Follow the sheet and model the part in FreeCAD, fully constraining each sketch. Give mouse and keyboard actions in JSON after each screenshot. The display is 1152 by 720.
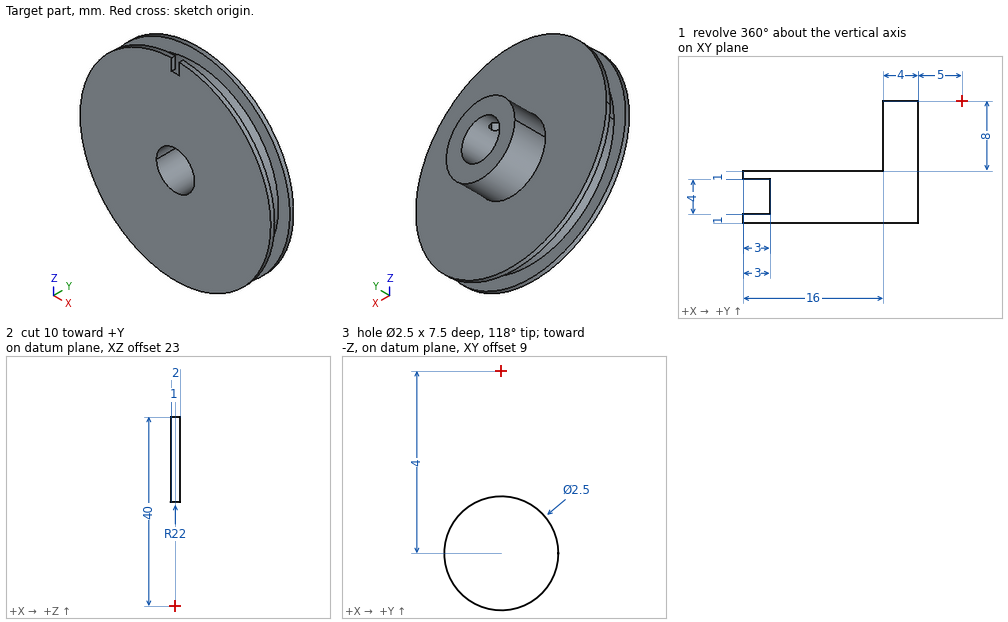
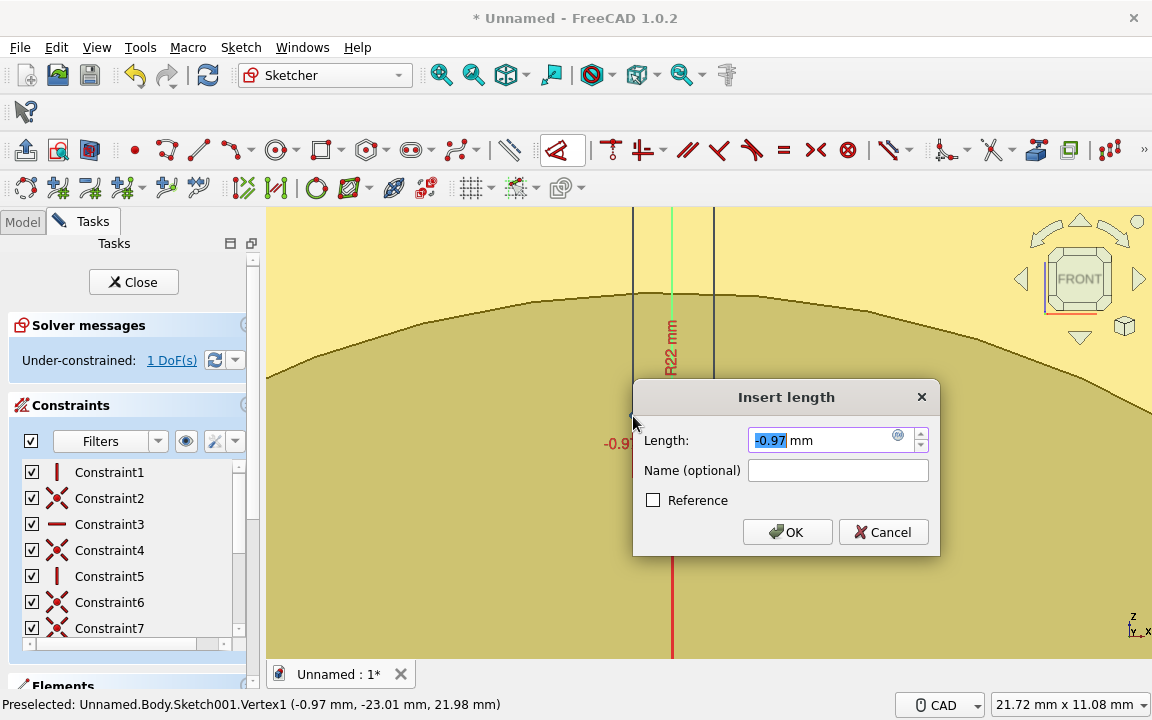
{"action": "type", "text": "-1"}
{"action": "key", "text": "Return"}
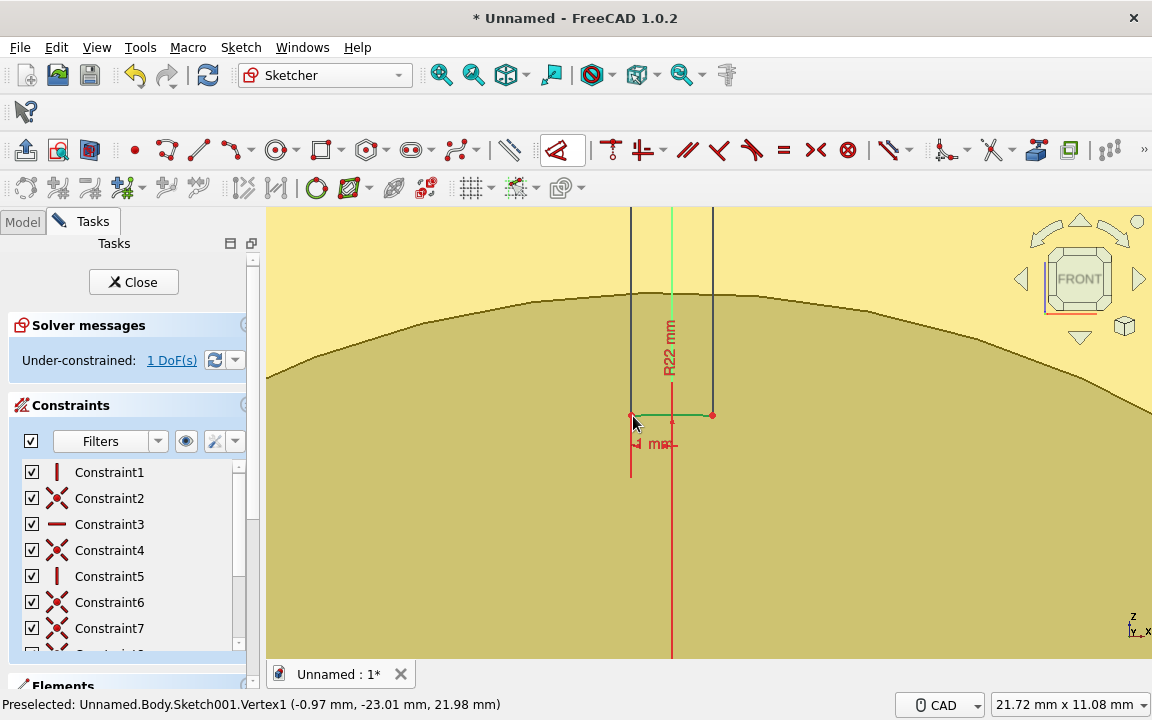
{"action": "scroll", "coordinate": [634, 420], "scroll_direction": "down", "scroll_amount": 9}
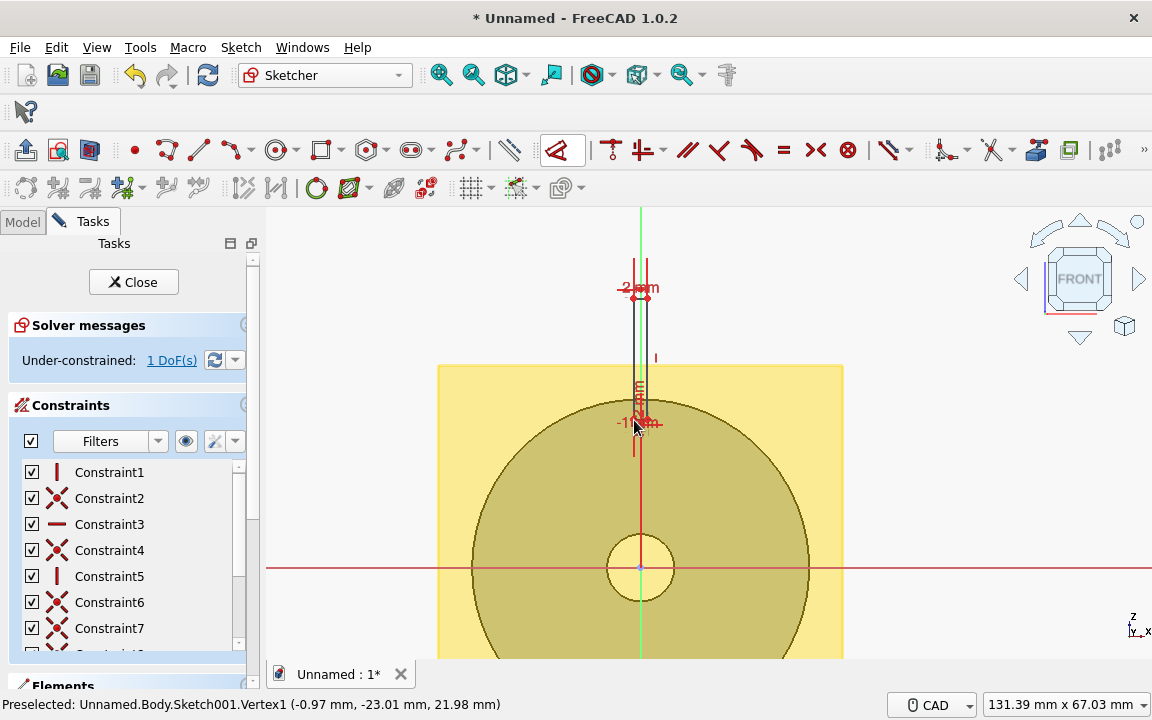
{"action": "left_click", "coordinate": [634, 299]}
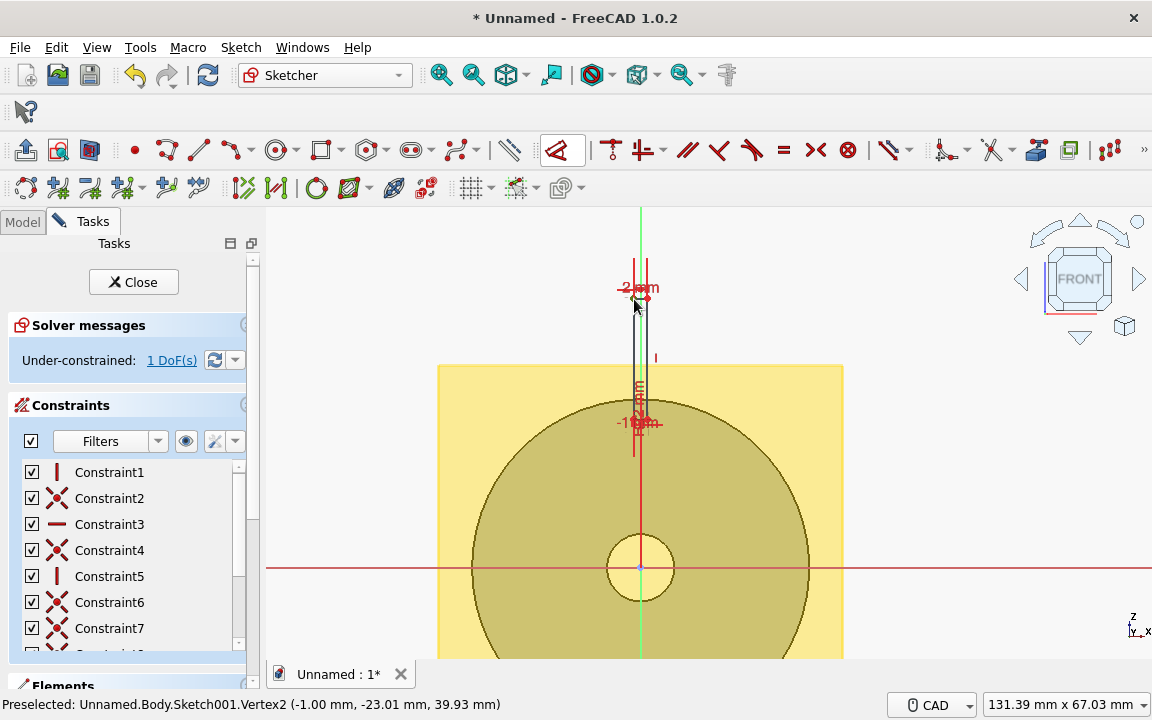
{"action": "left_click", "coordinate": [580, 150]}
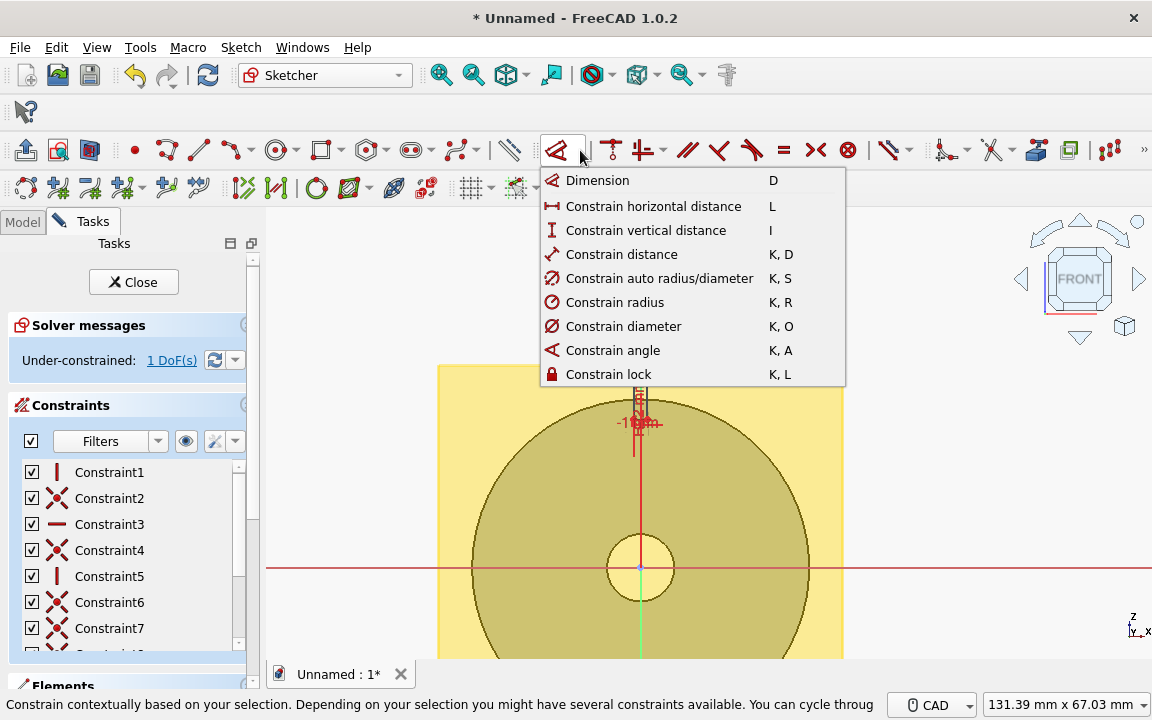
{"action": "left_click", "coordinate": [693, 230]}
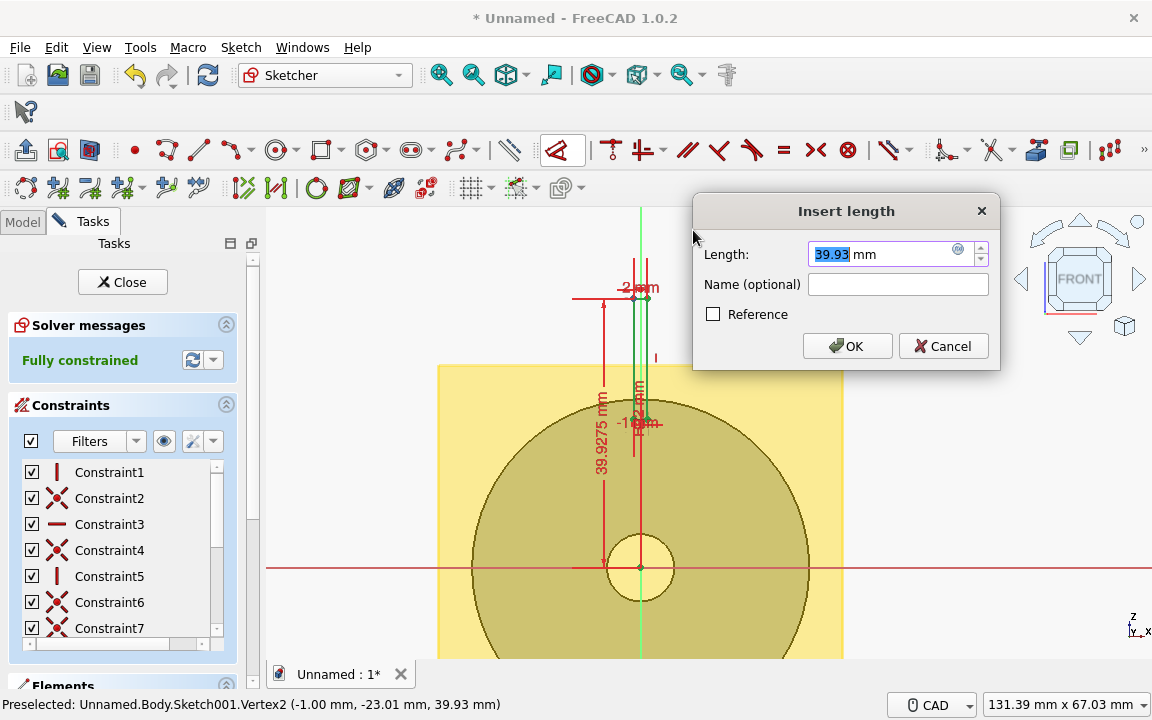
{"action": "type", "text": "40"}
{"action": "key", "text": "Return"}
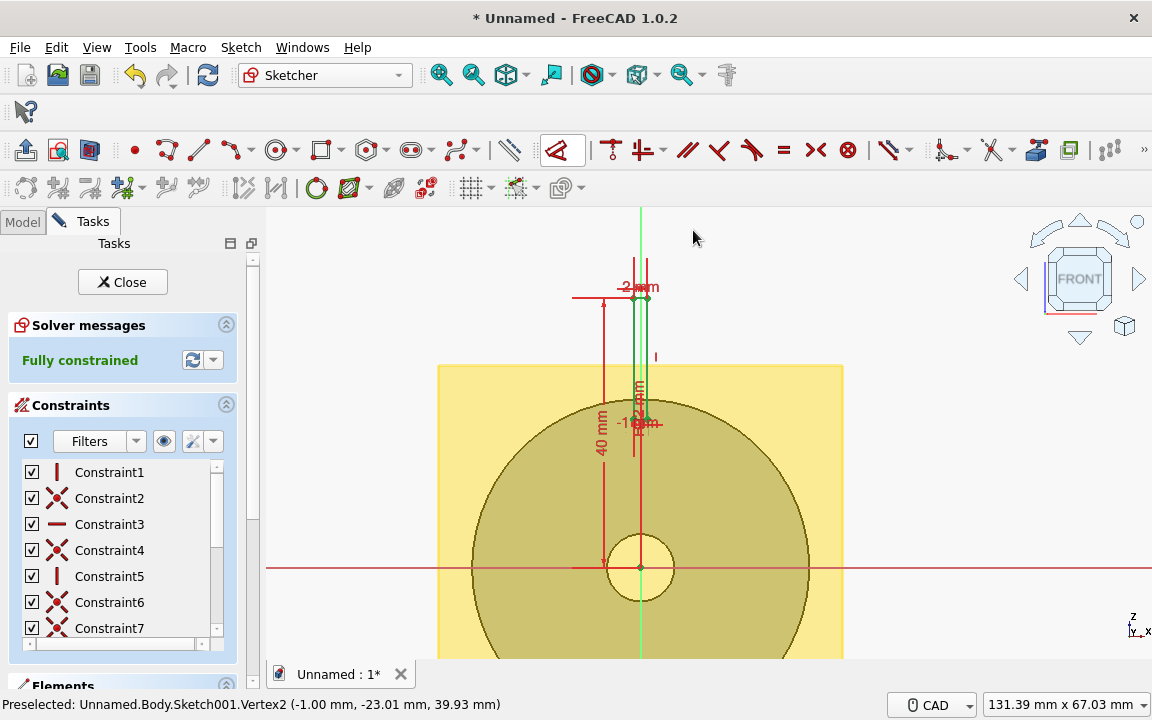
{"action": "left_click", "coordinate": [123, 282]}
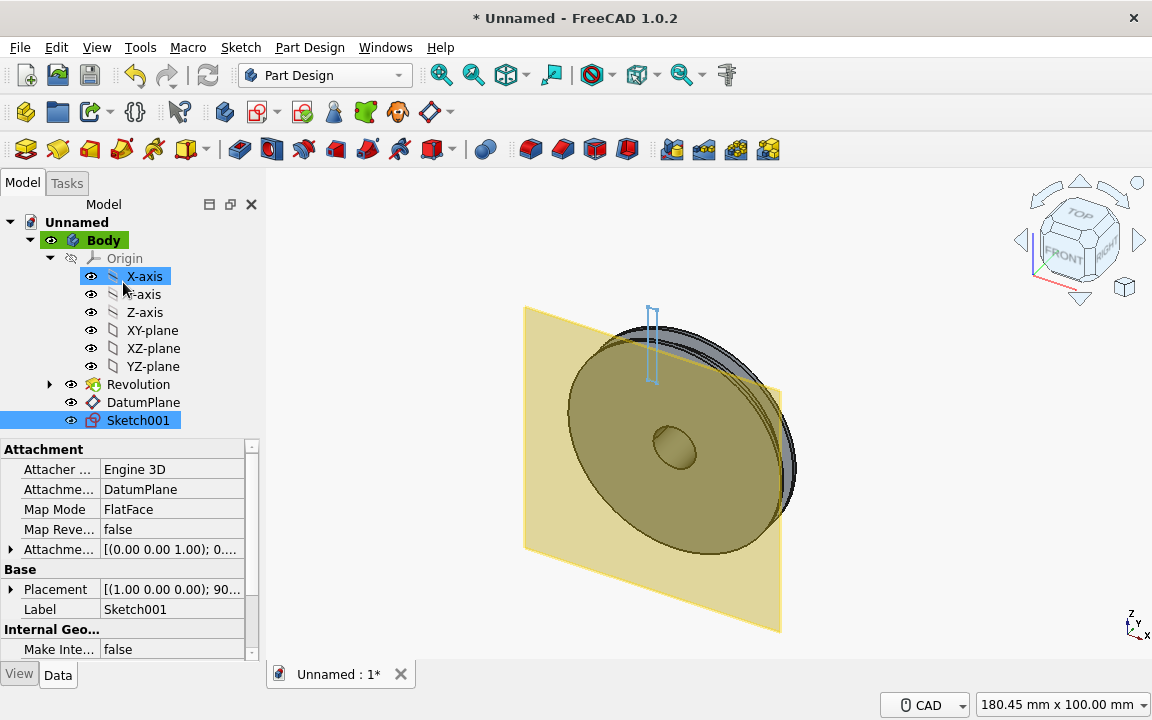
{"action": "left_click", "coordinate": [240, 150]}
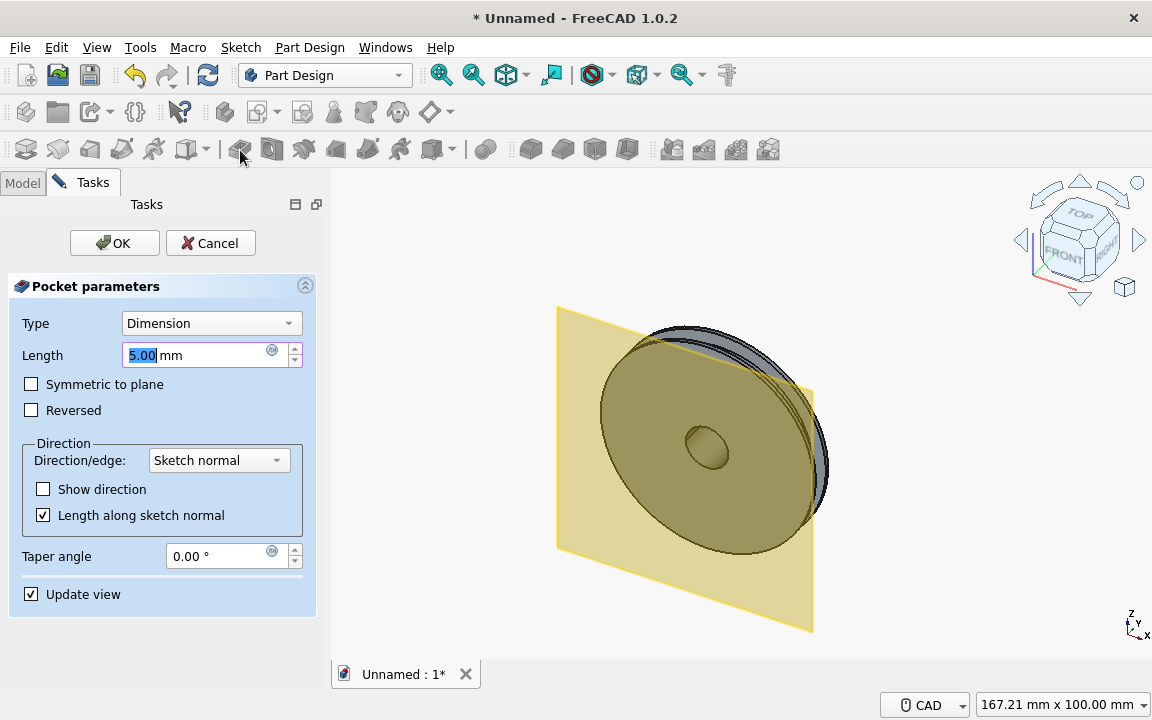
{"action": "type", "text": "10"}
{"action": "key", "text": "Tab"}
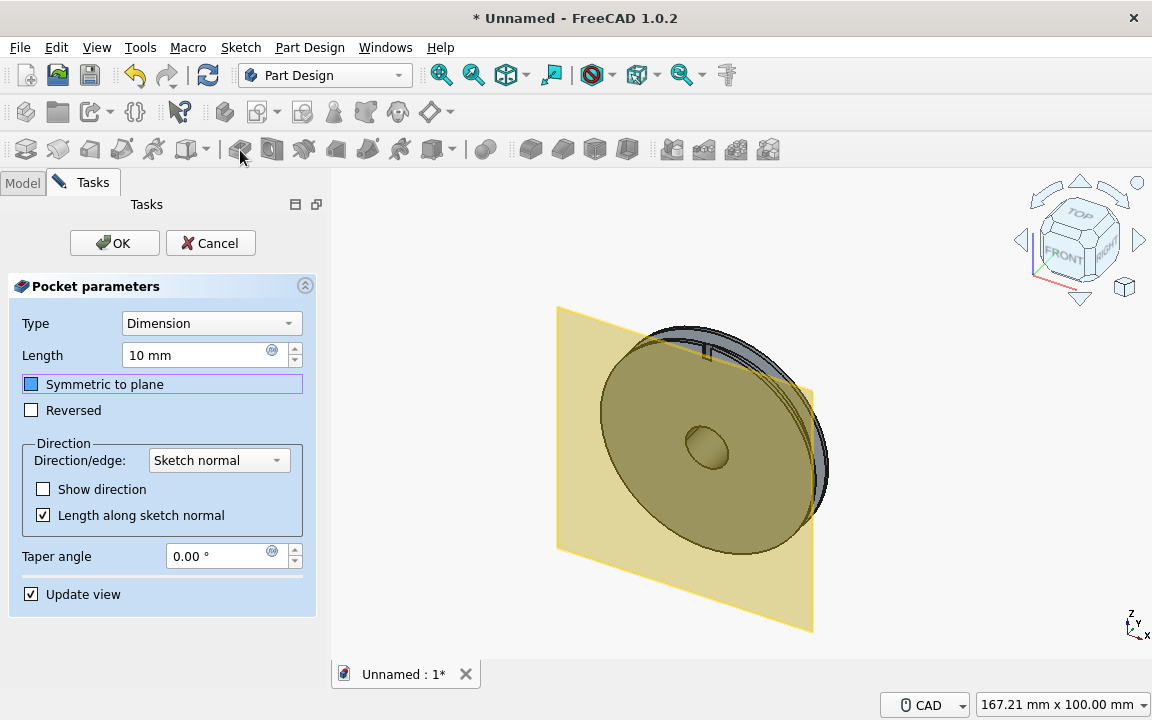
{"action": "left_click", "coordinate": [115, 243]}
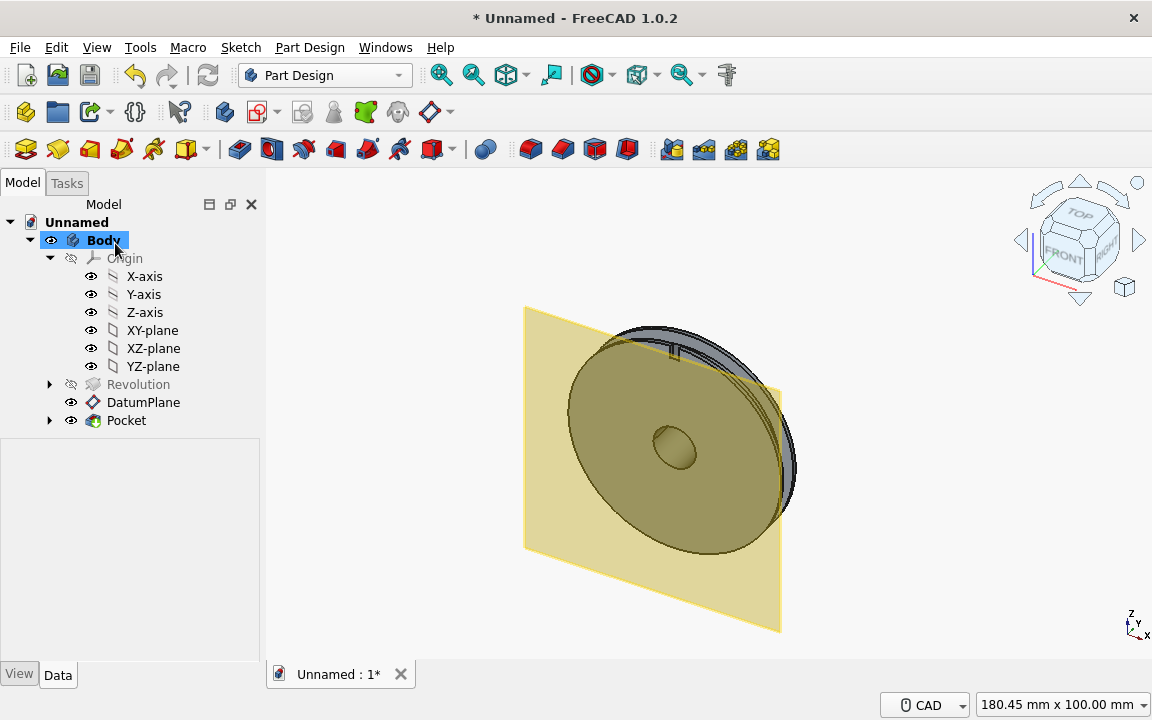
{"action": "left_click", "coordinate": [116, 402]}
{"action": "key", "text": "space"}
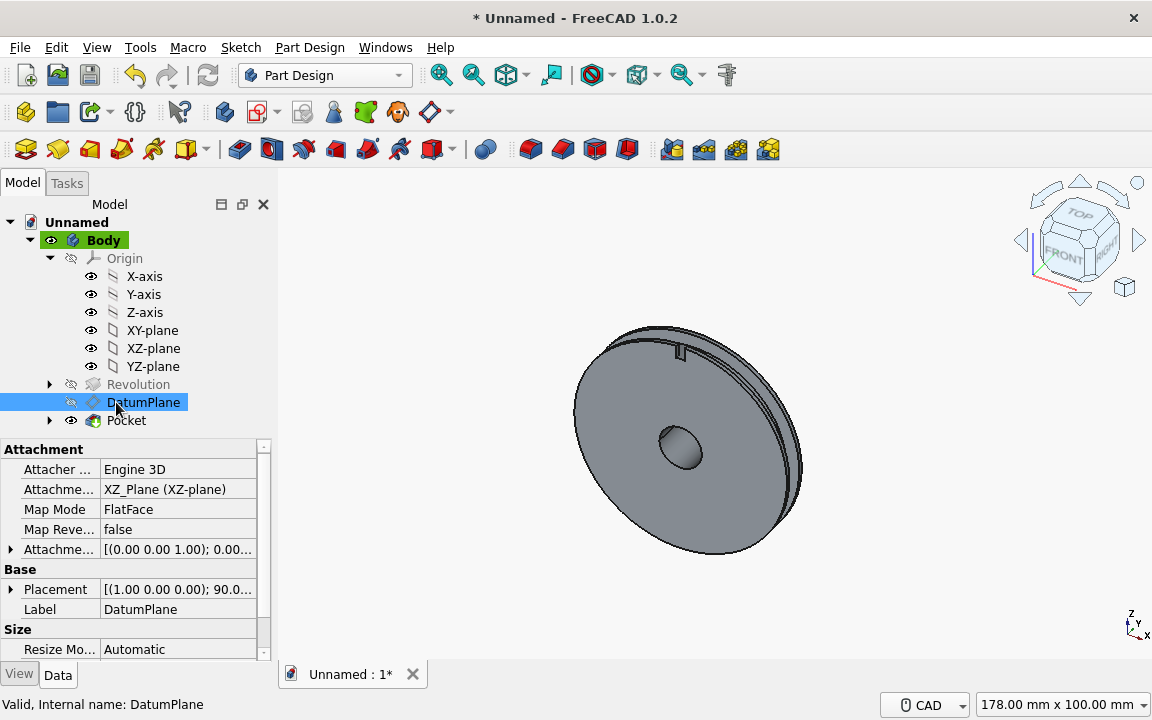
{"action": "left_click", "coordinate": [136, 330]}